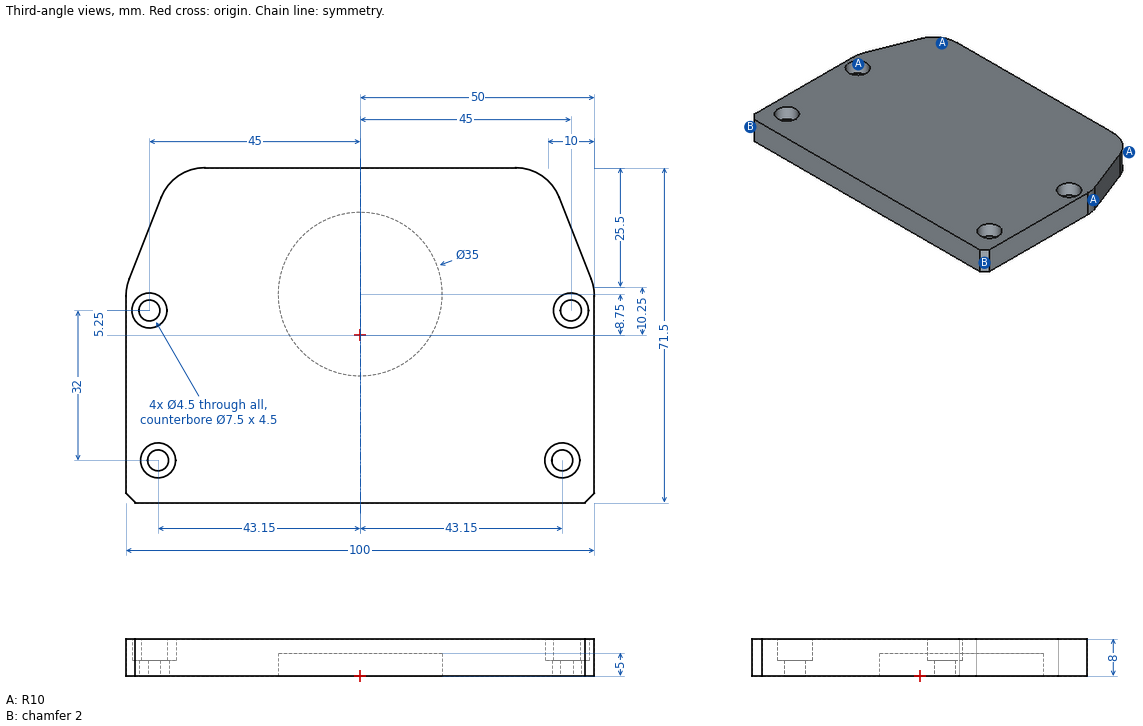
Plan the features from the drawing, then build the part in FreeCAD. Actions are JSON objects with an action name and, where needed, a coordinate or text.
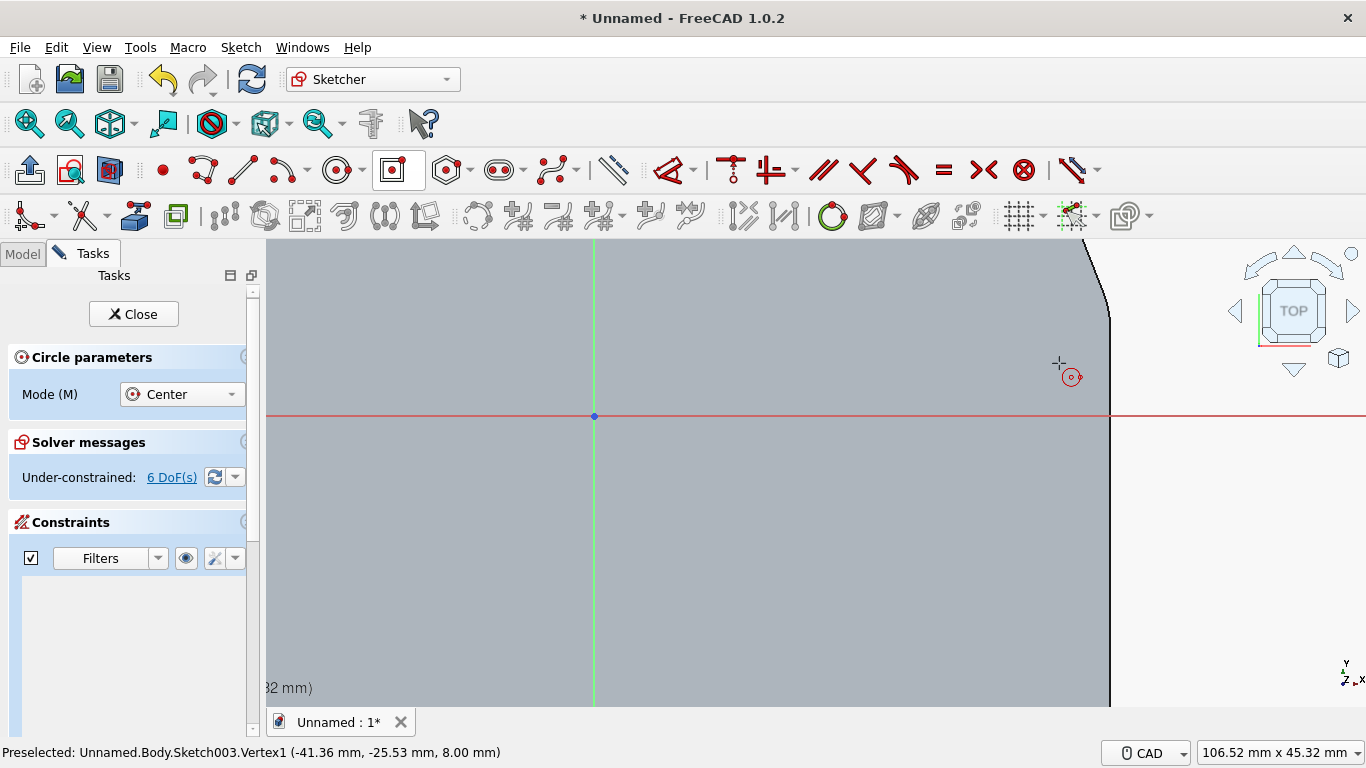
{"action": "left_click", "coordinate": [1059, 362]}
{"action": "left_click", "coordinate": [1075, 346]}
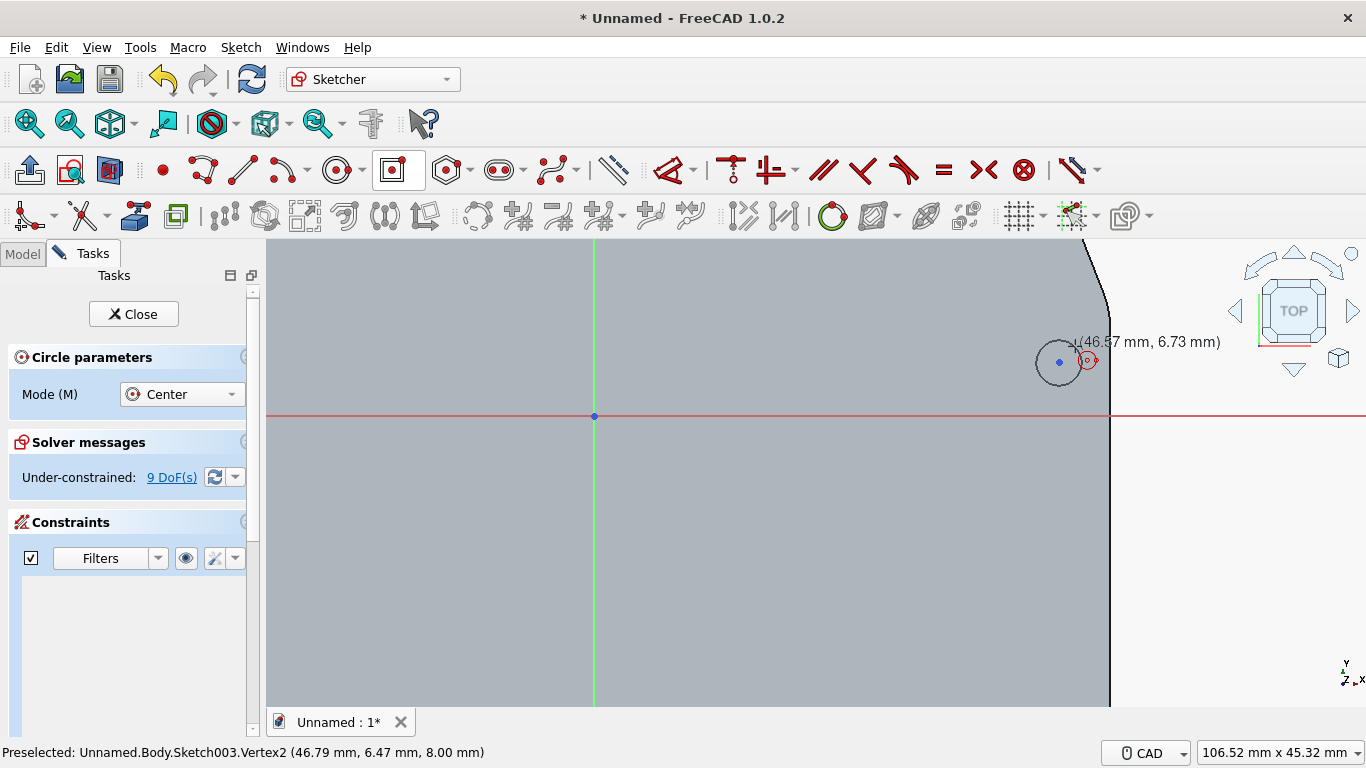
{"action": "scroll", "coordinate": [1059, 362], "scroll_direction": "down", "scroll_amount": 2}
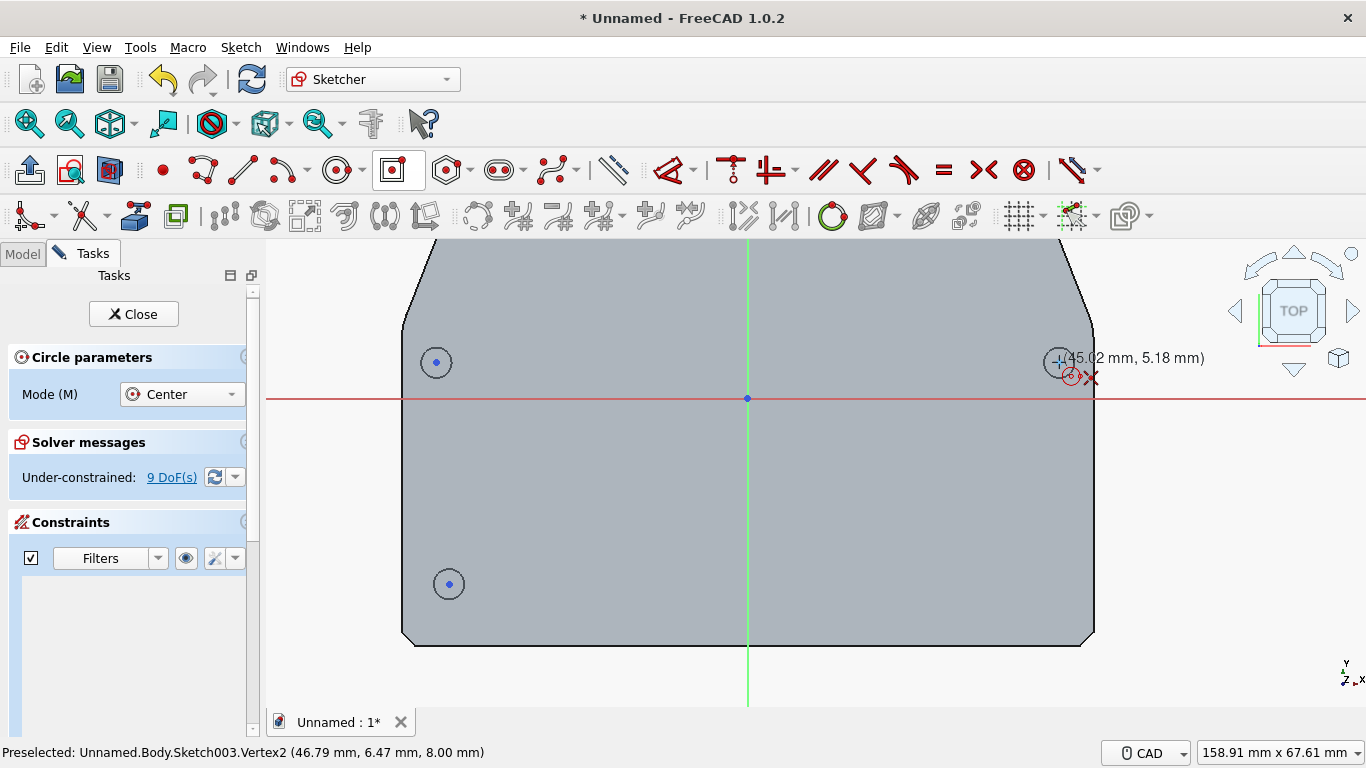
{"action": "scroll", "coordinate": [1046, 584], "scroll_direction": "up", "scroll_amount": 2}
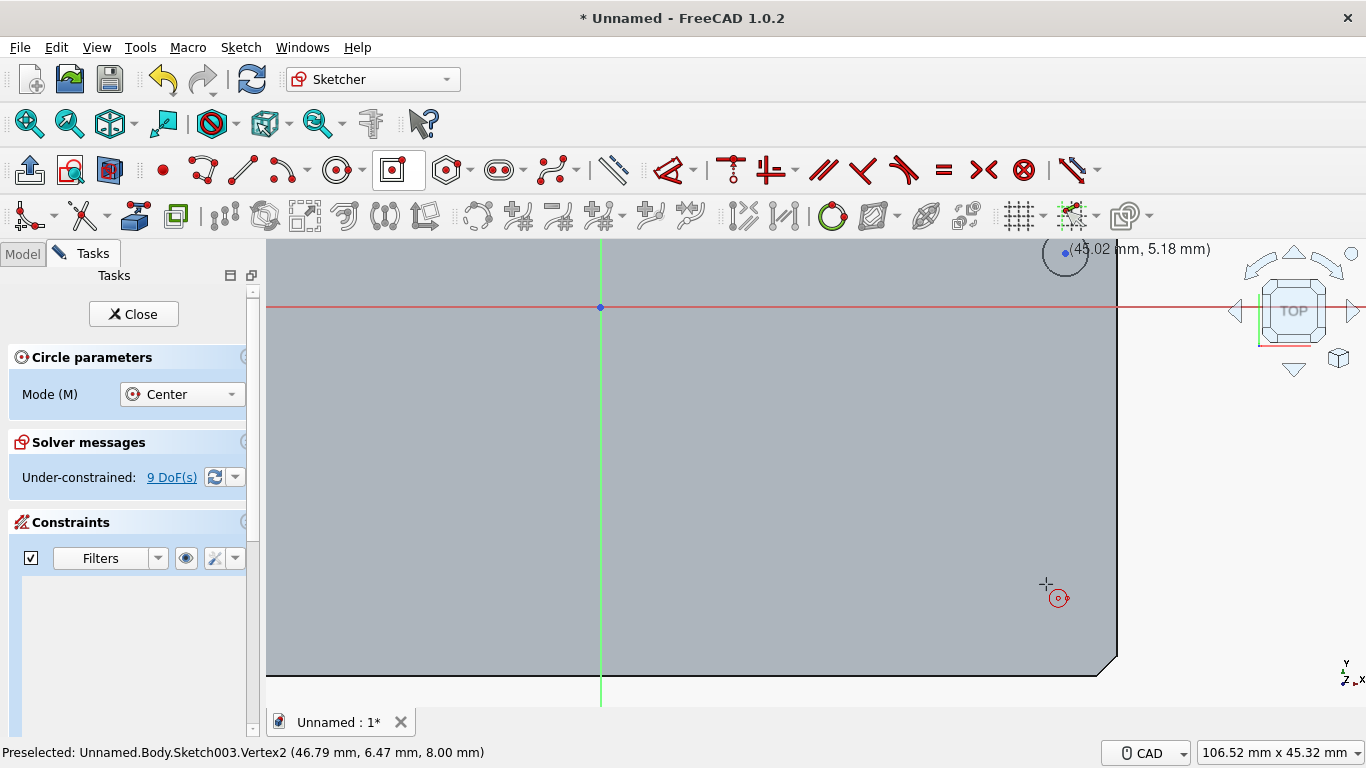
{"action": "left_click", "coordinate": [1046, 583]}
{"action": "left_click", "coordinate": [1063, 567]}
{"action": "key", "text": "Escape"}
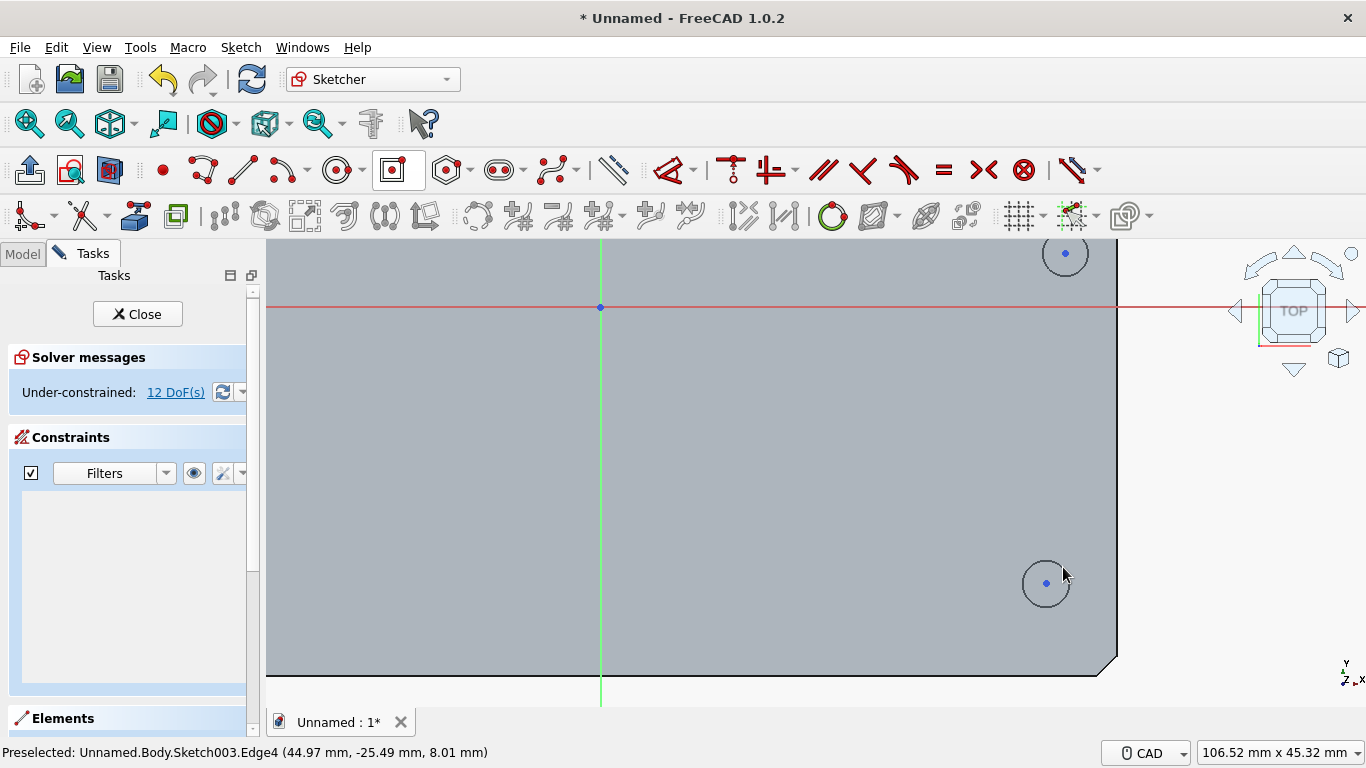
{"action": "scroll", "coordinate": [1046, 585], "scroll_direction": "down", "scroll_amount": 2}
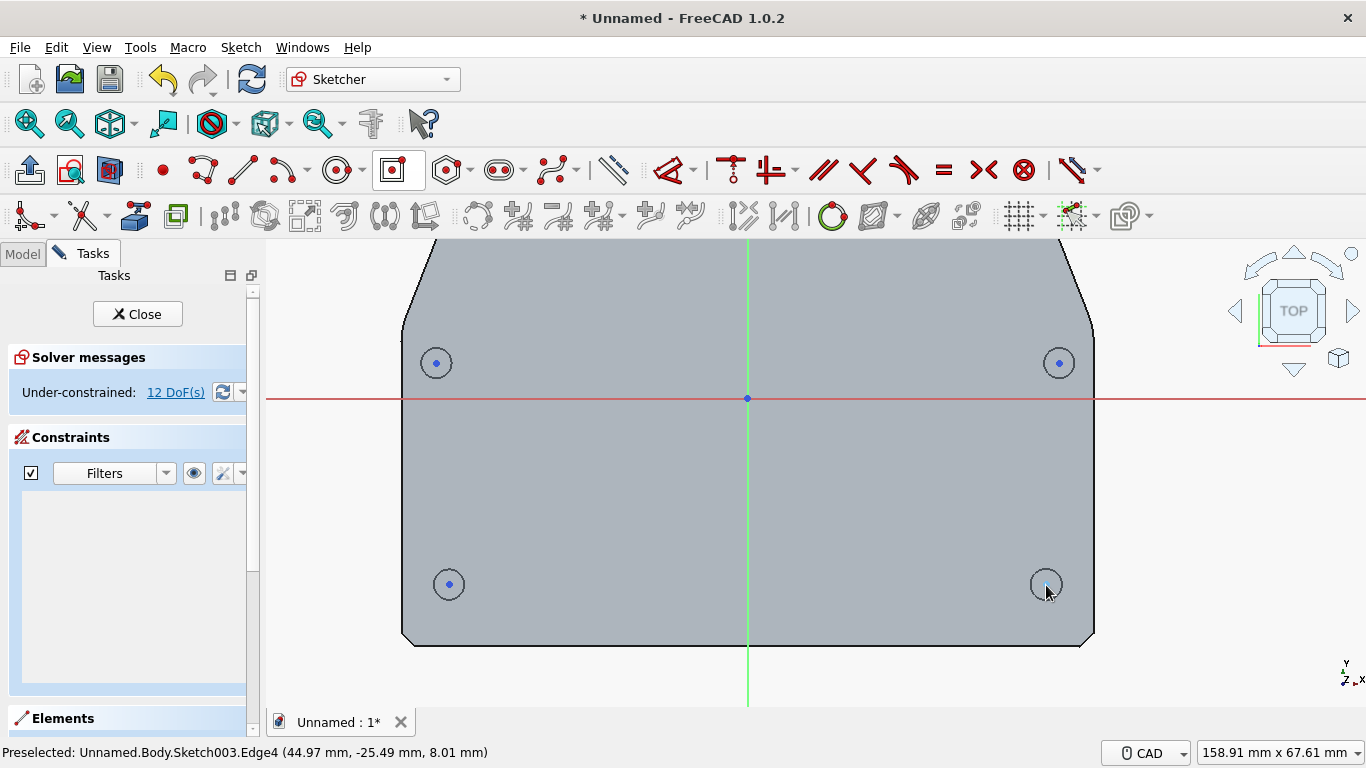
{"action": "left_click", "coordinate": [447, 352]}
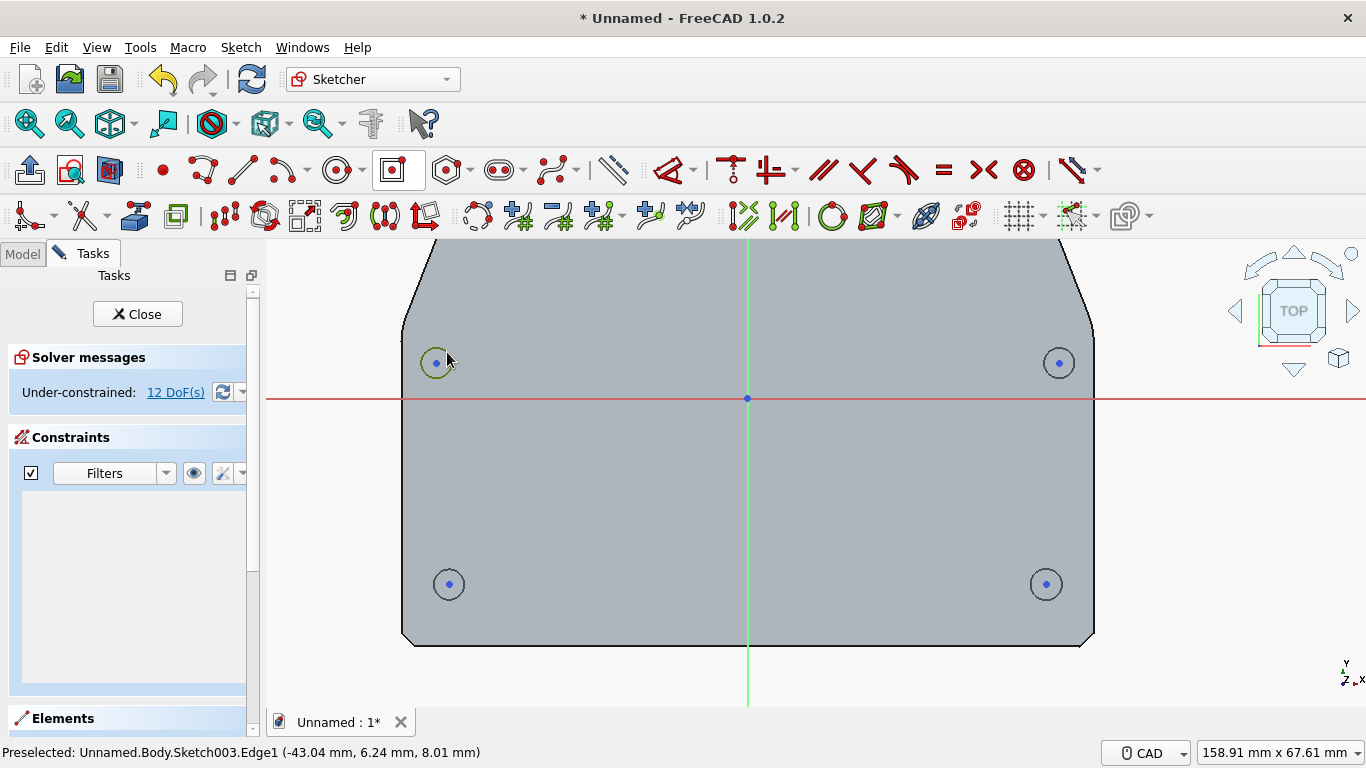
{"action": "left_click", "coordinate": [460, 574]}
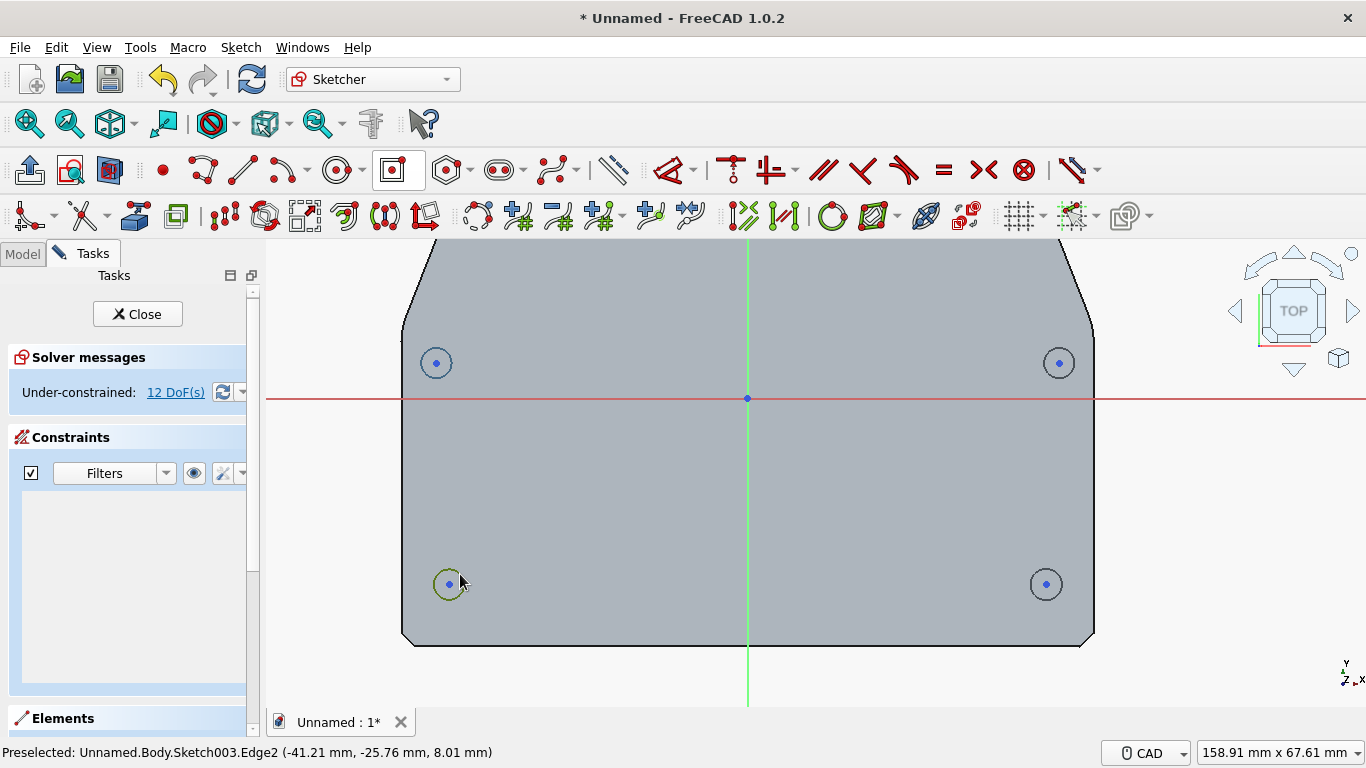
{"action": "left_click", "coordinate": [1070, 352]}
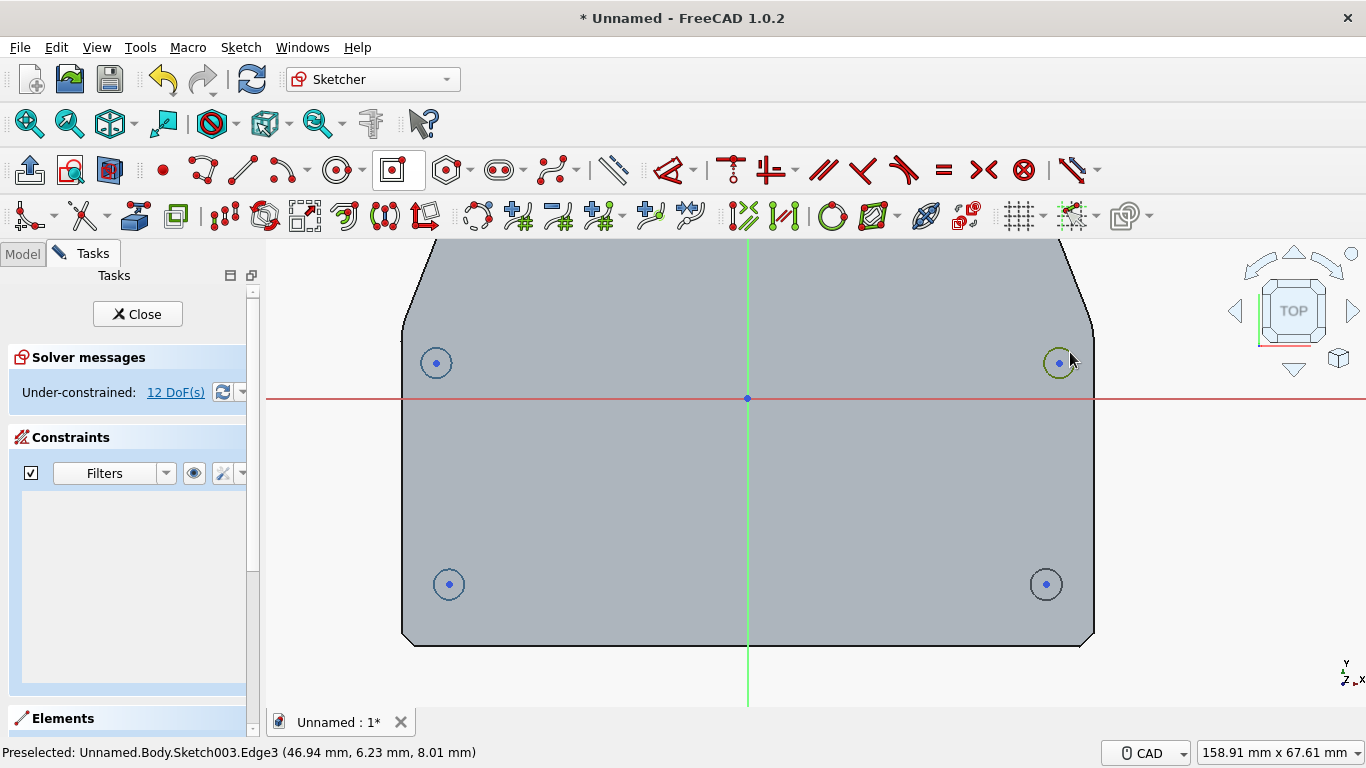
{"action": "left_click", "coordinate": [1057, 573]}